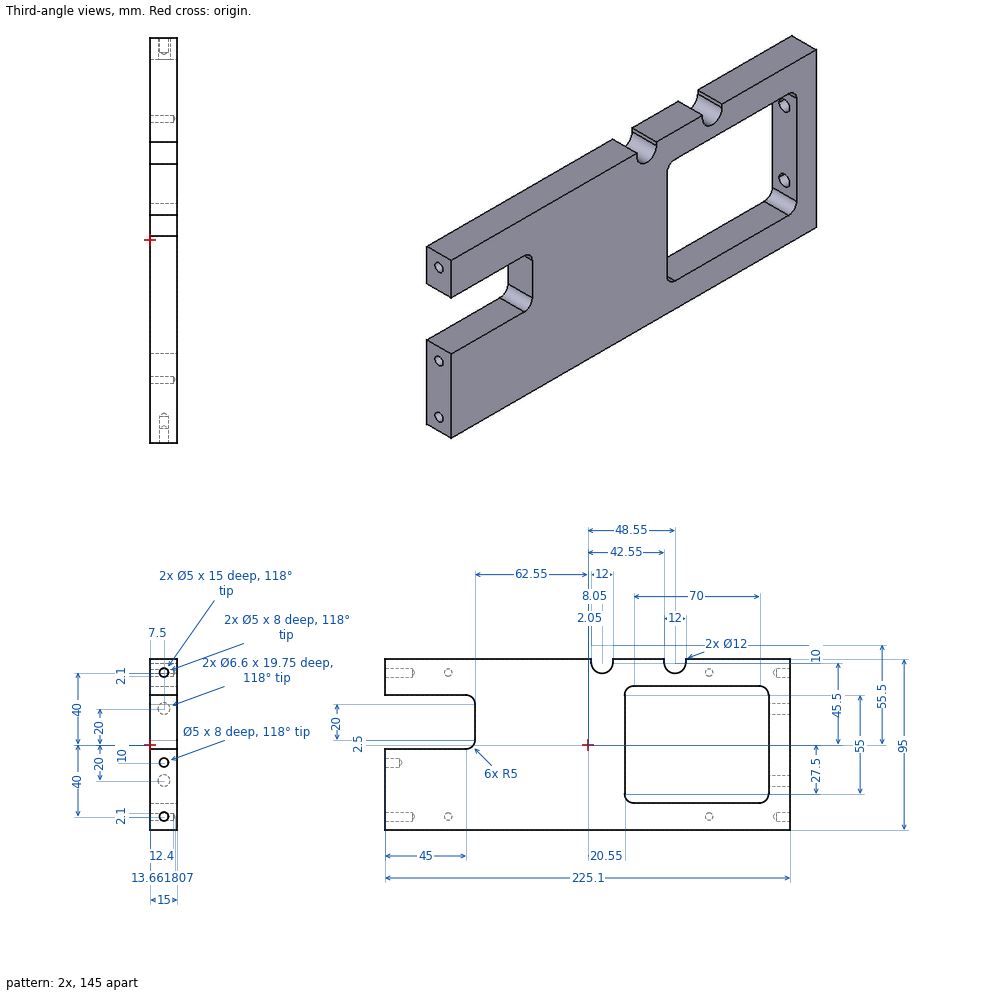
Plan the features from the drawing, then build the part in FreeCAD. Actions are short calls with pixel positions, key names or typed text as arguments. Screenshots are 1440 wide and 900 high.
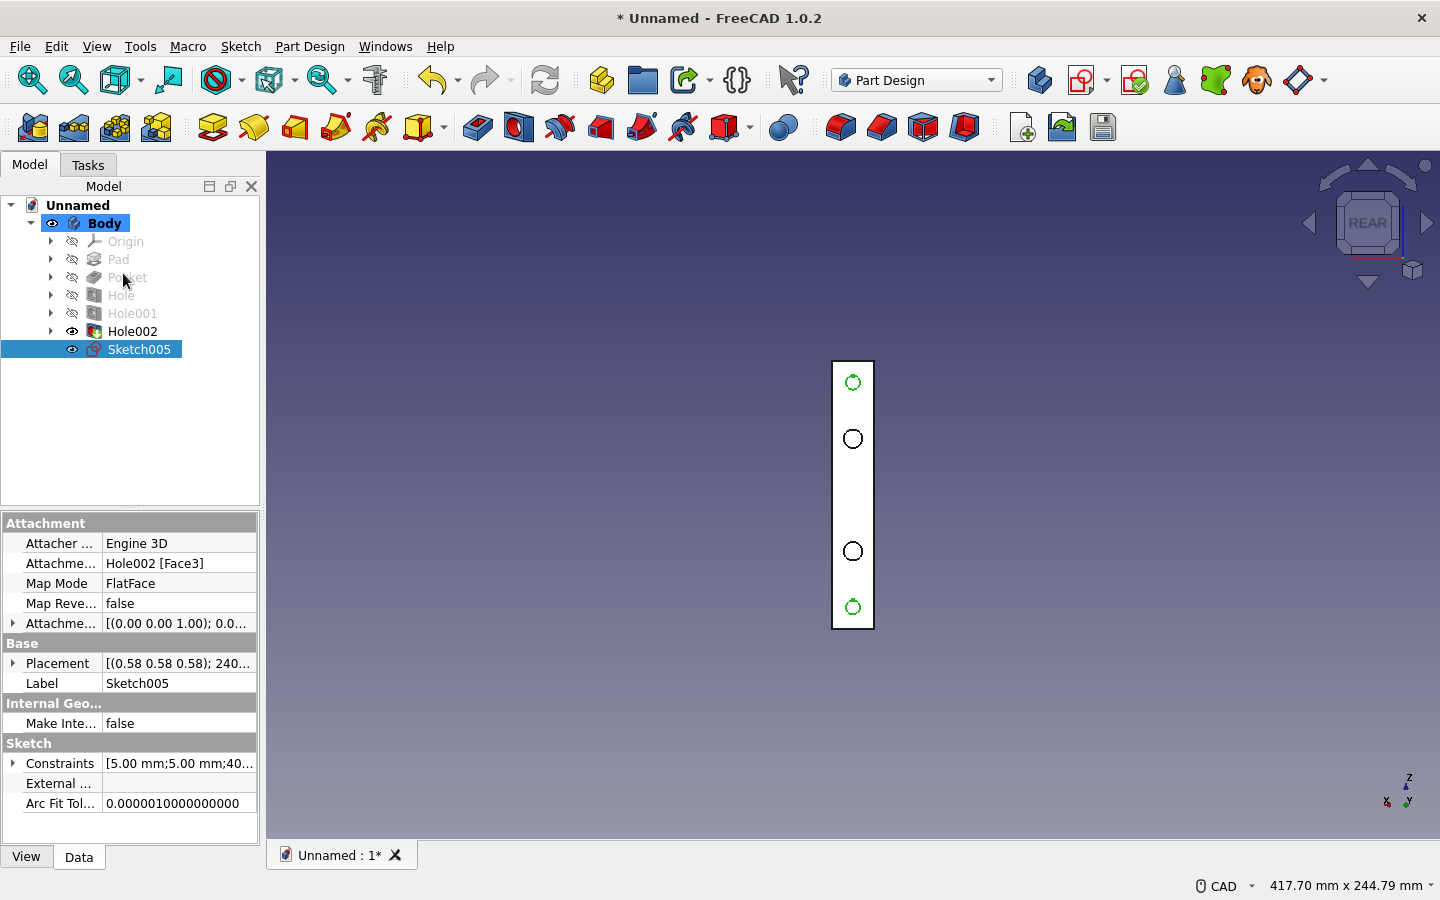
click(519, 128)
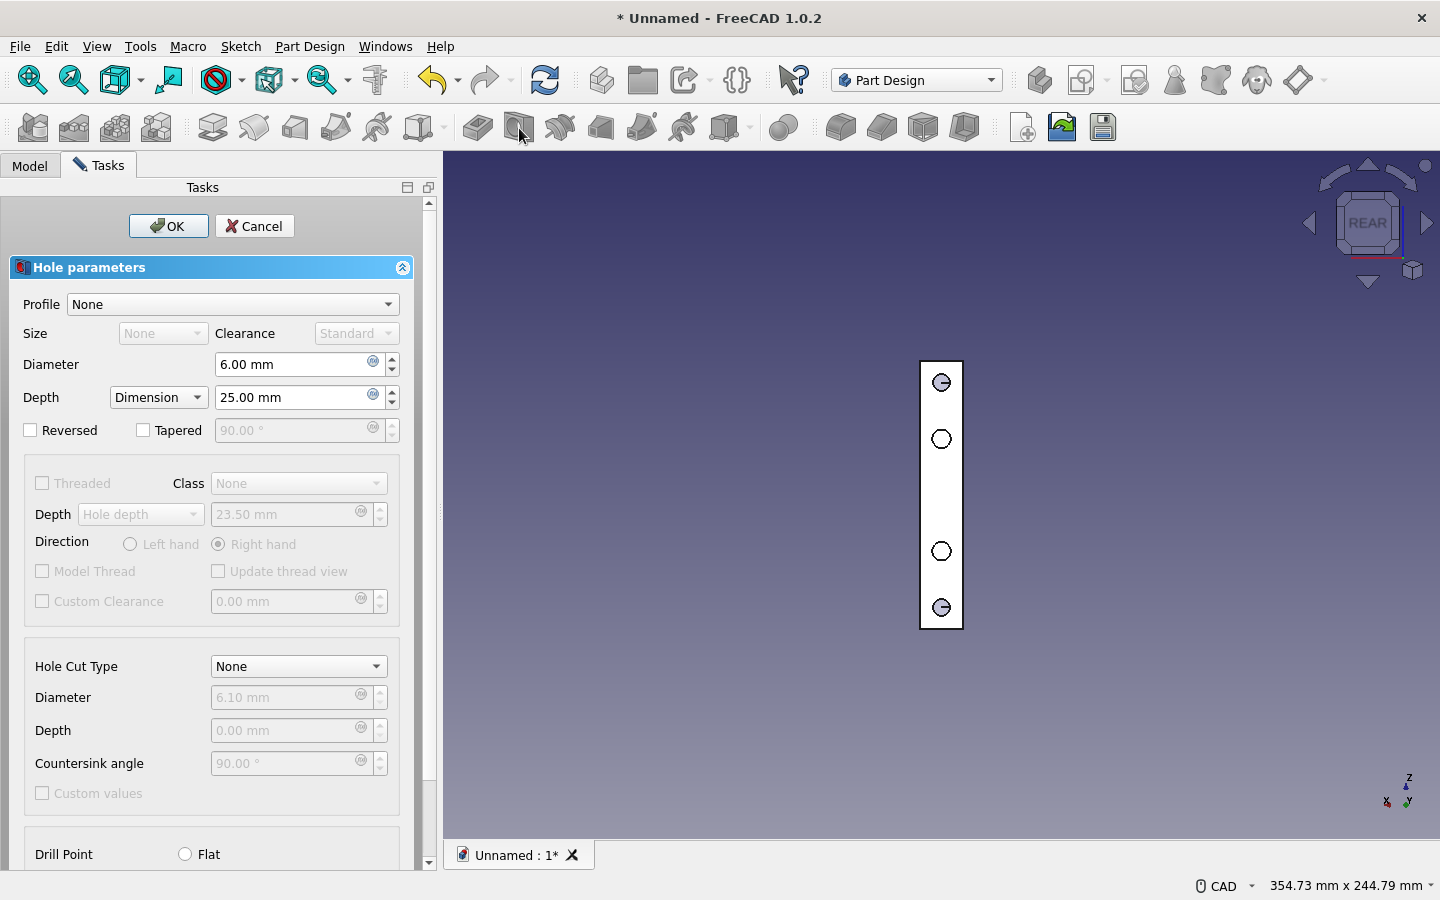
triple_click(300, 364)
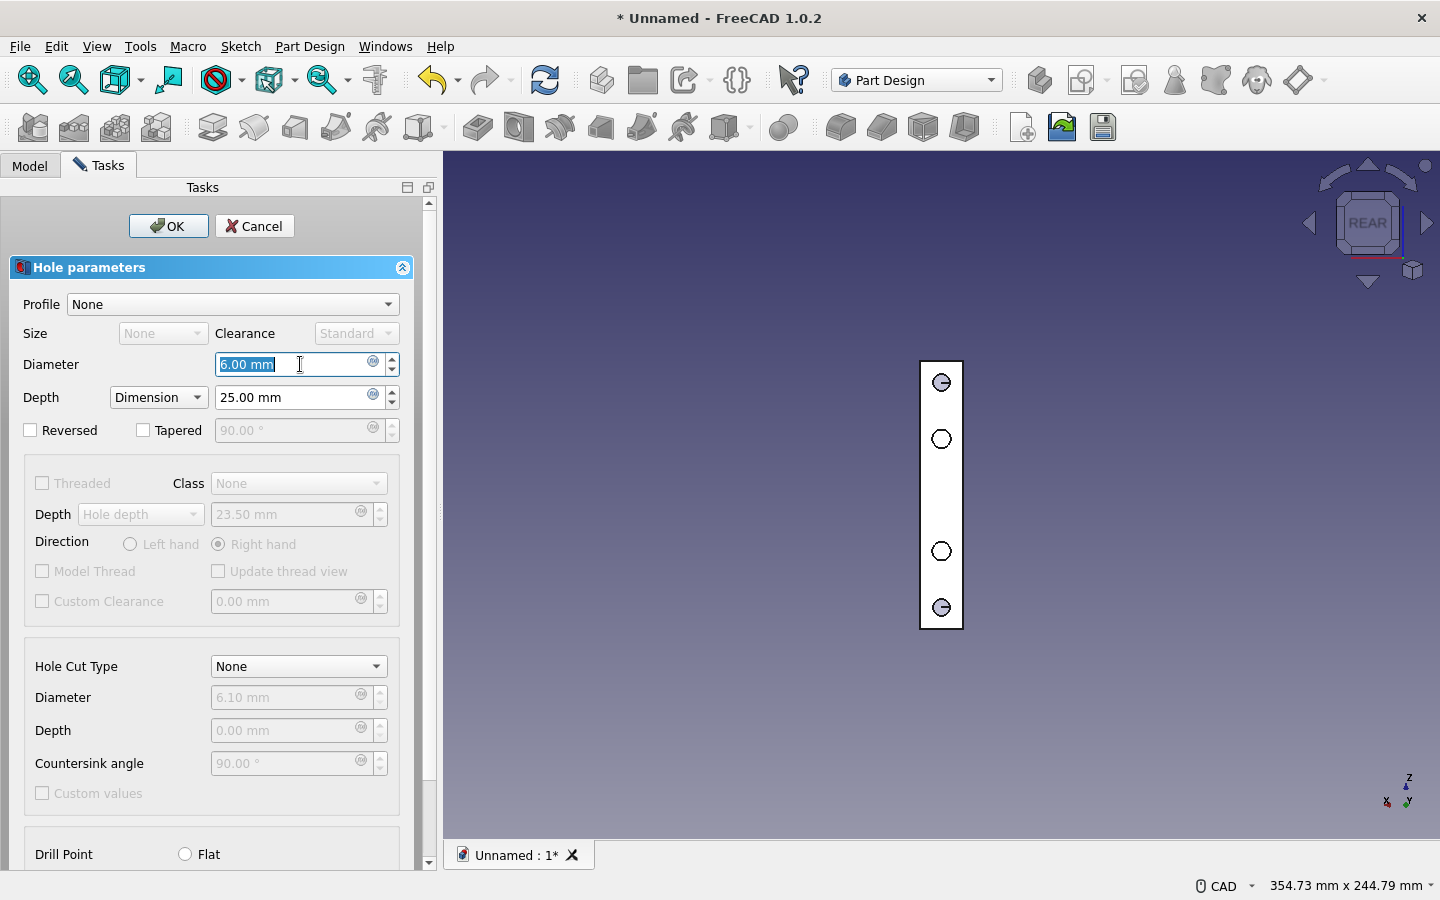
text(5)
key(Tab)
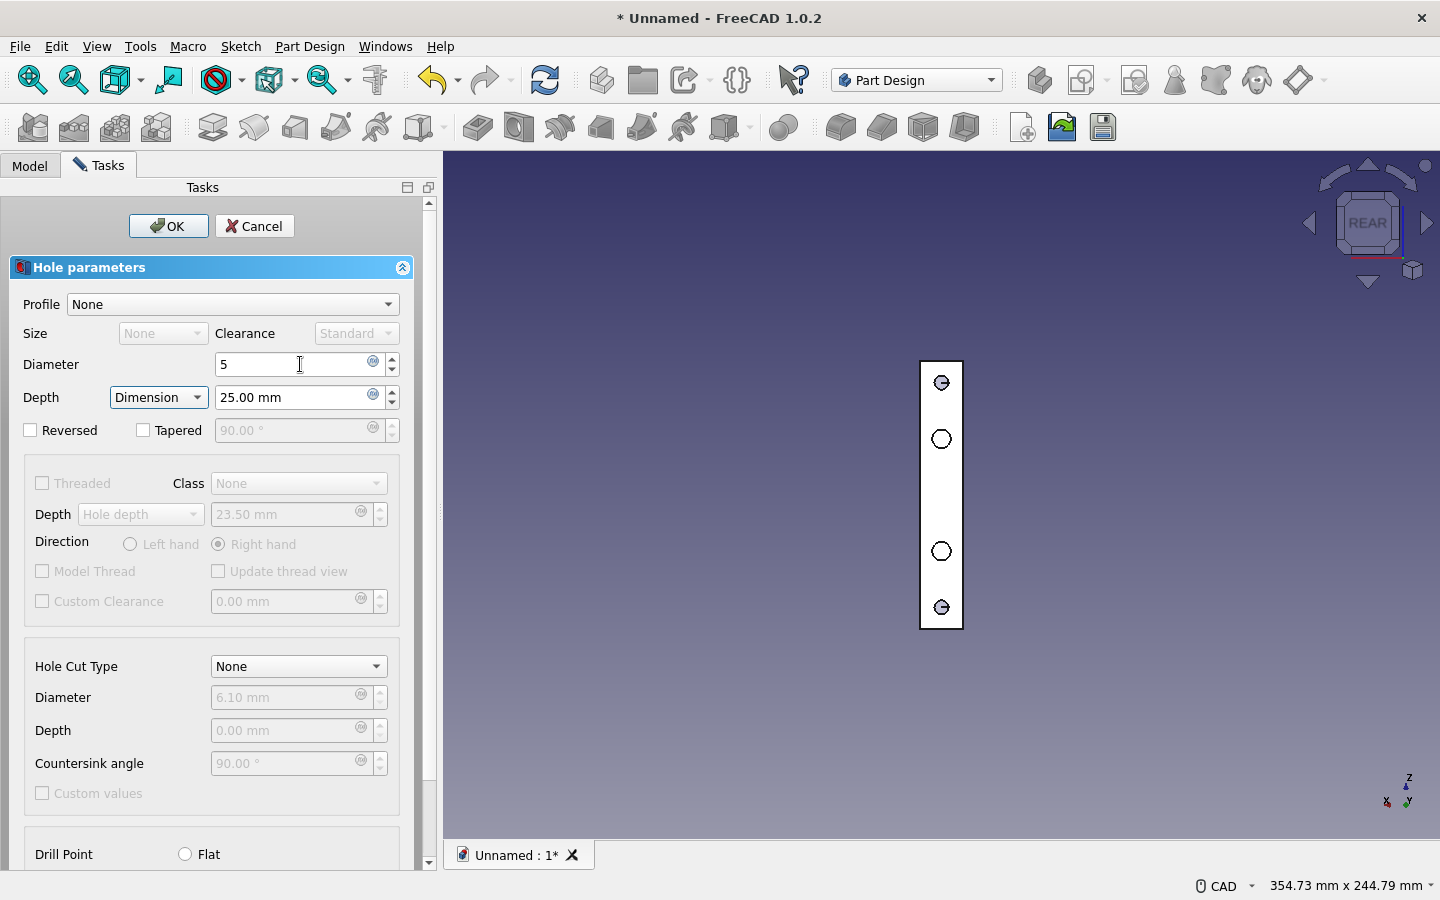
triple_click(300, 398)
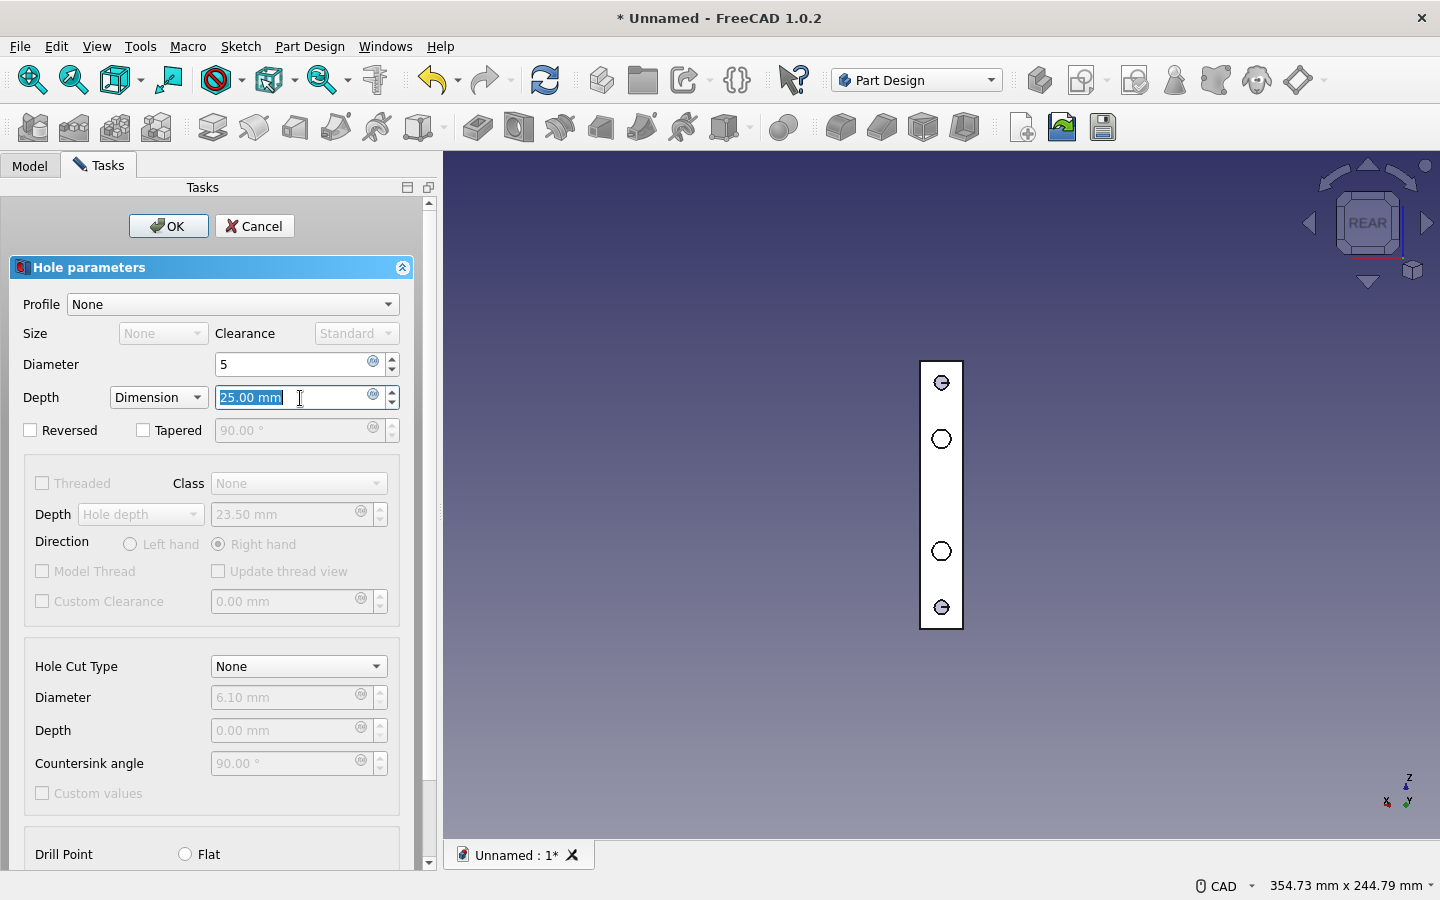
text(8)
key(Tab)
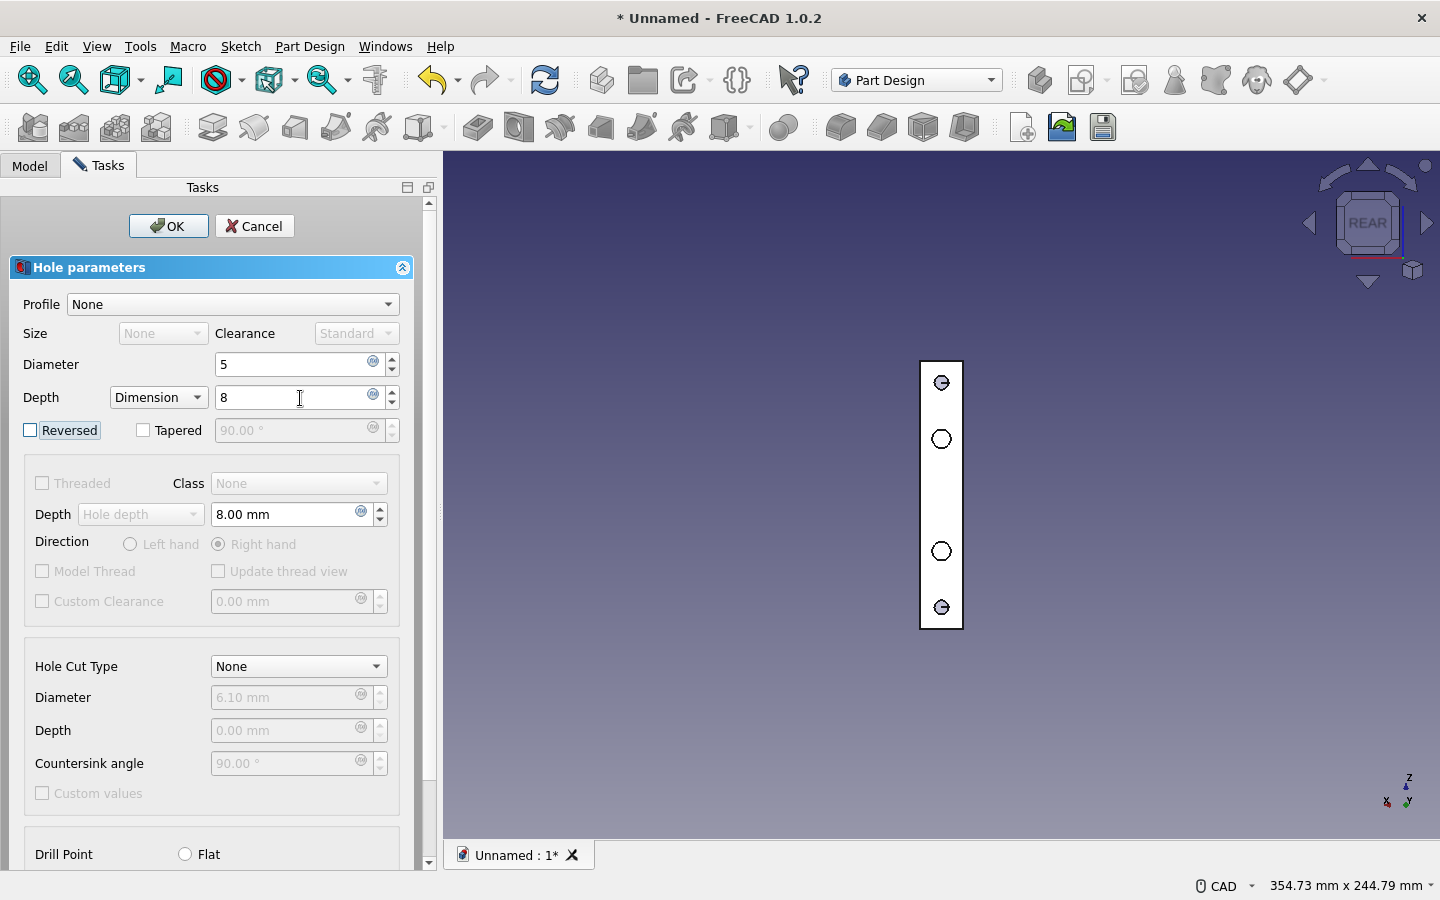
click(169, 226)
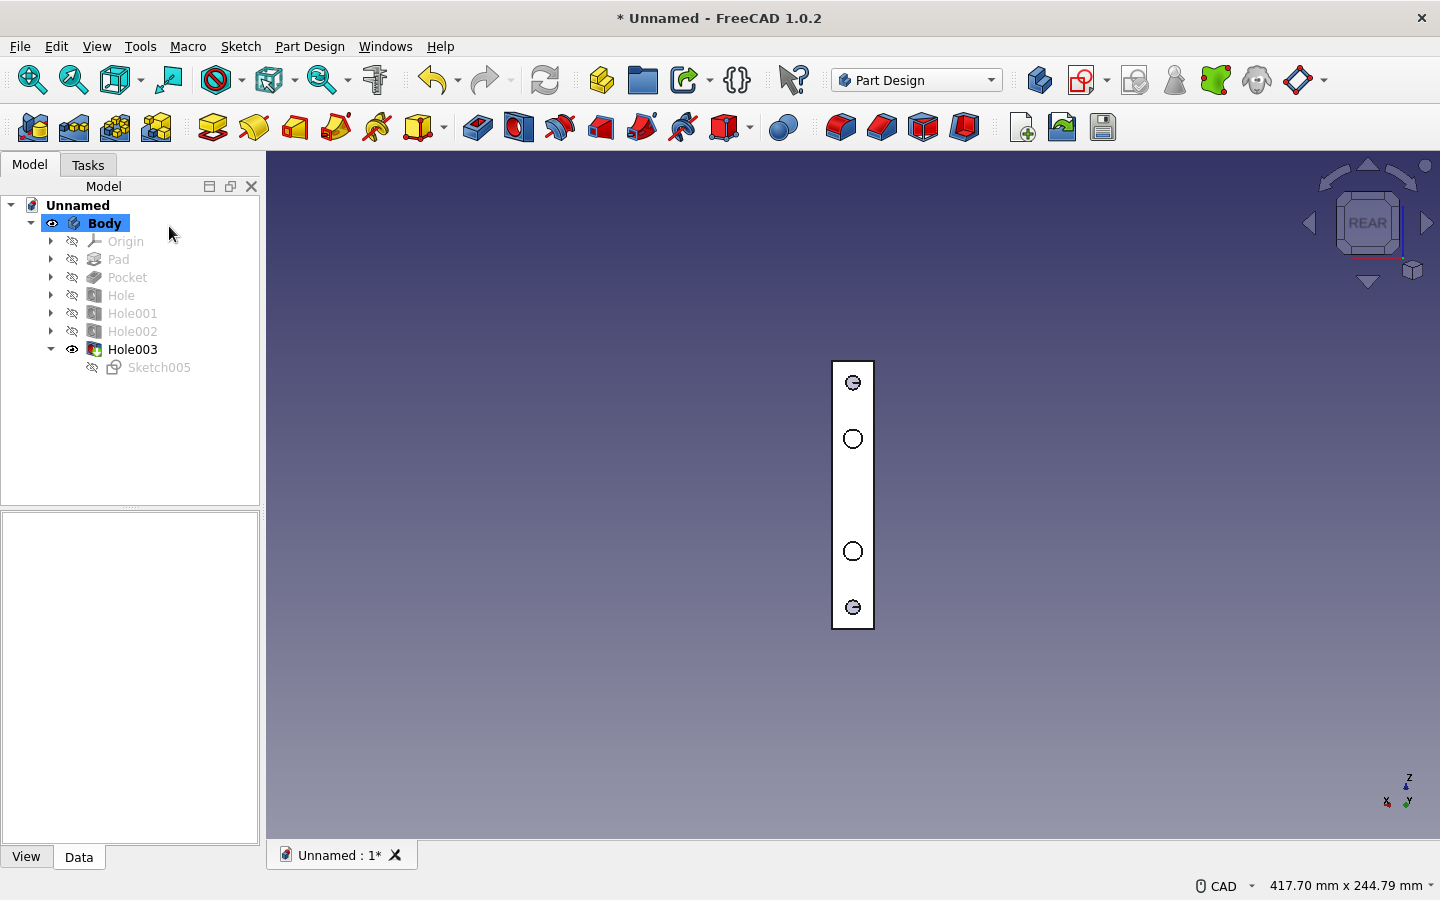
click(33, 80)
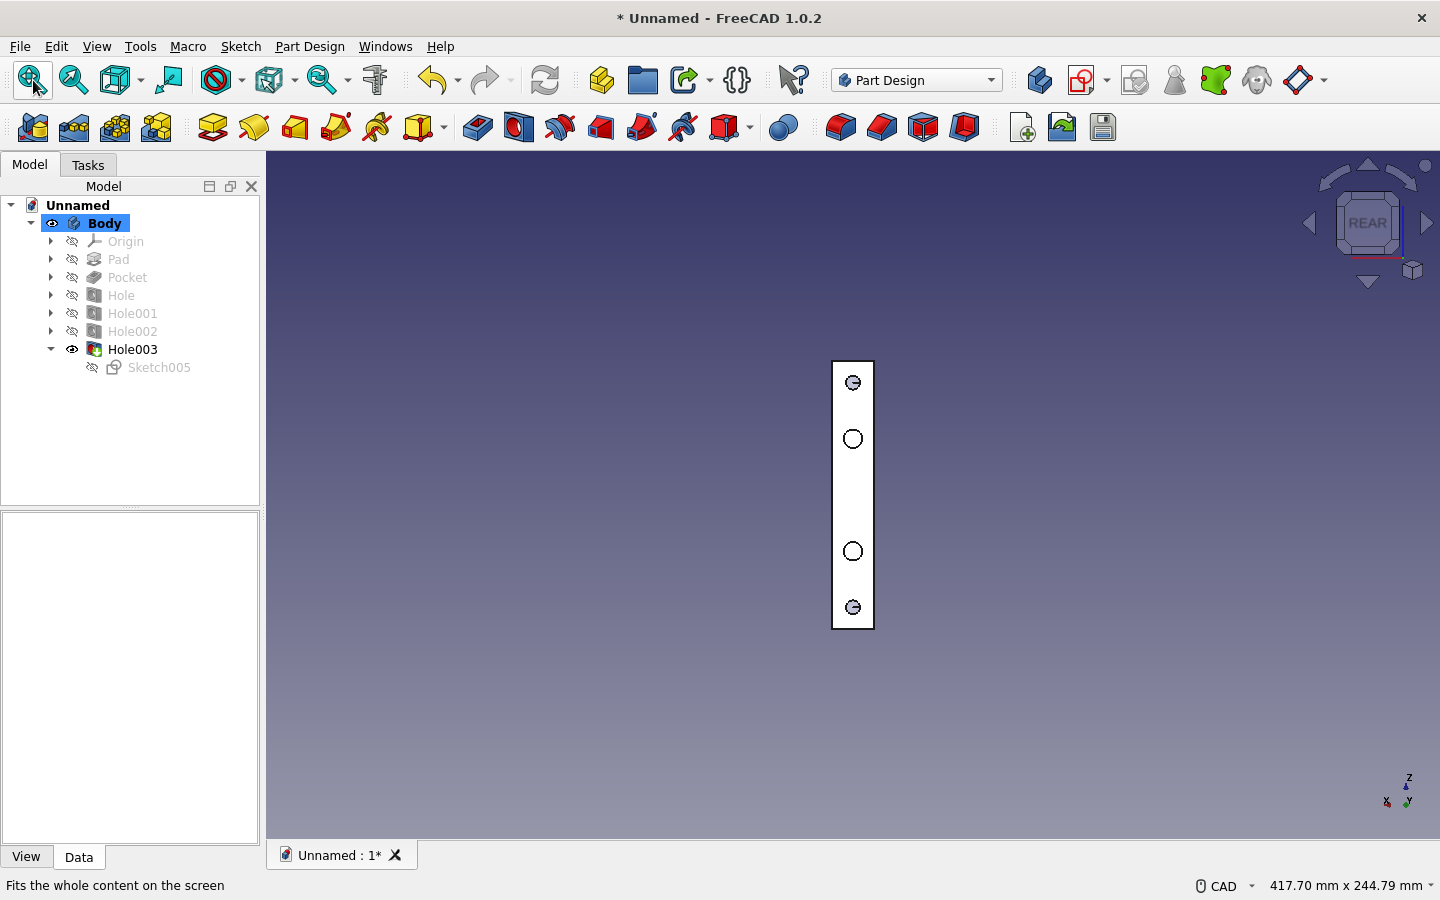
key(0)